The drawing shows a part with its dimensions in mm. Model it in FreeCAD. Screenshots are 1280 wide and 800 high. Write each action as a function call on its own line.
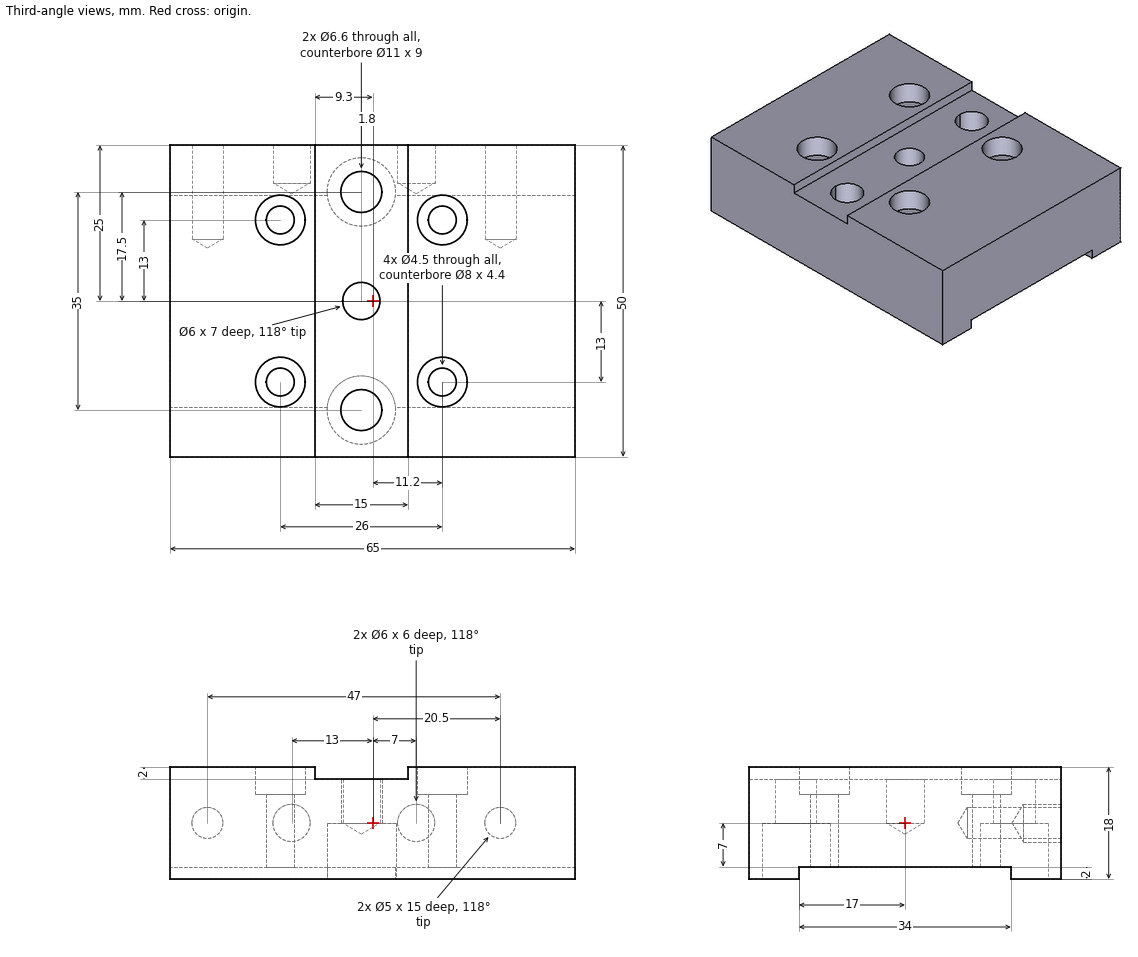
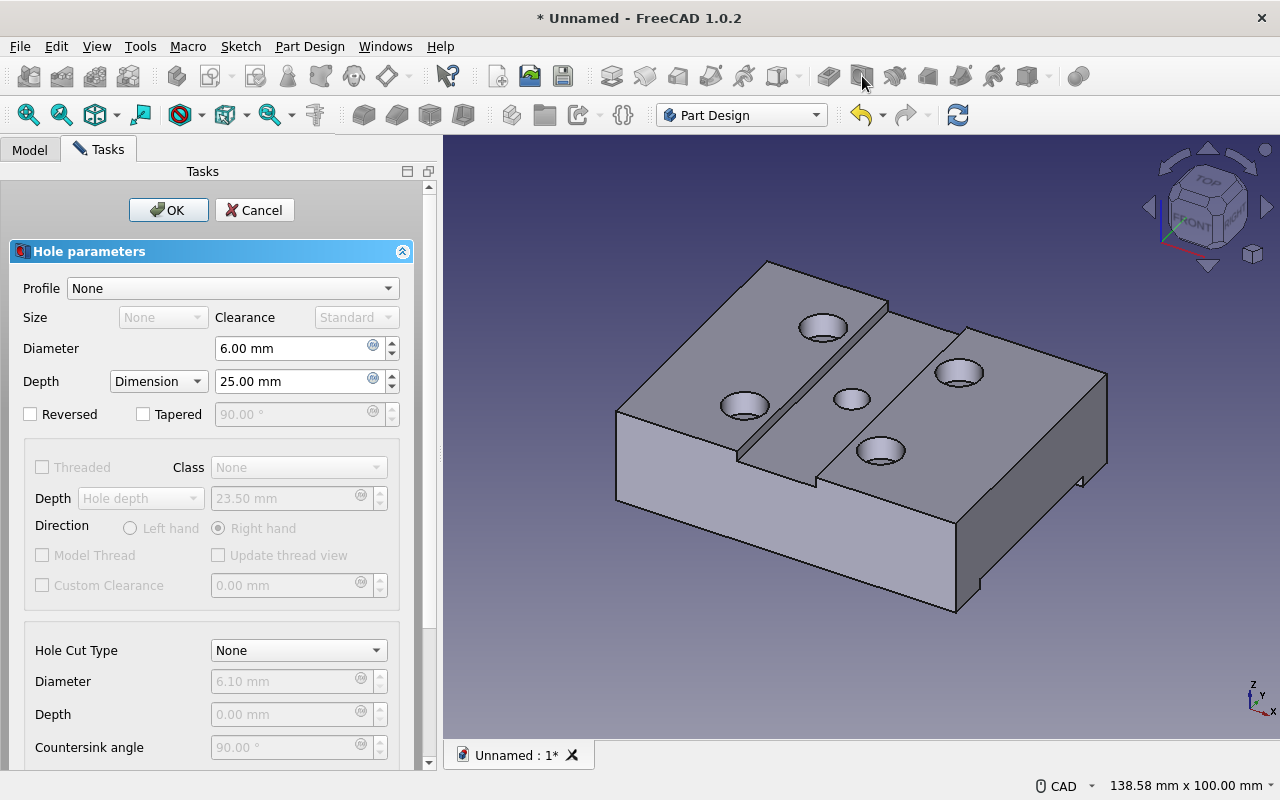
triple_click(300, 348)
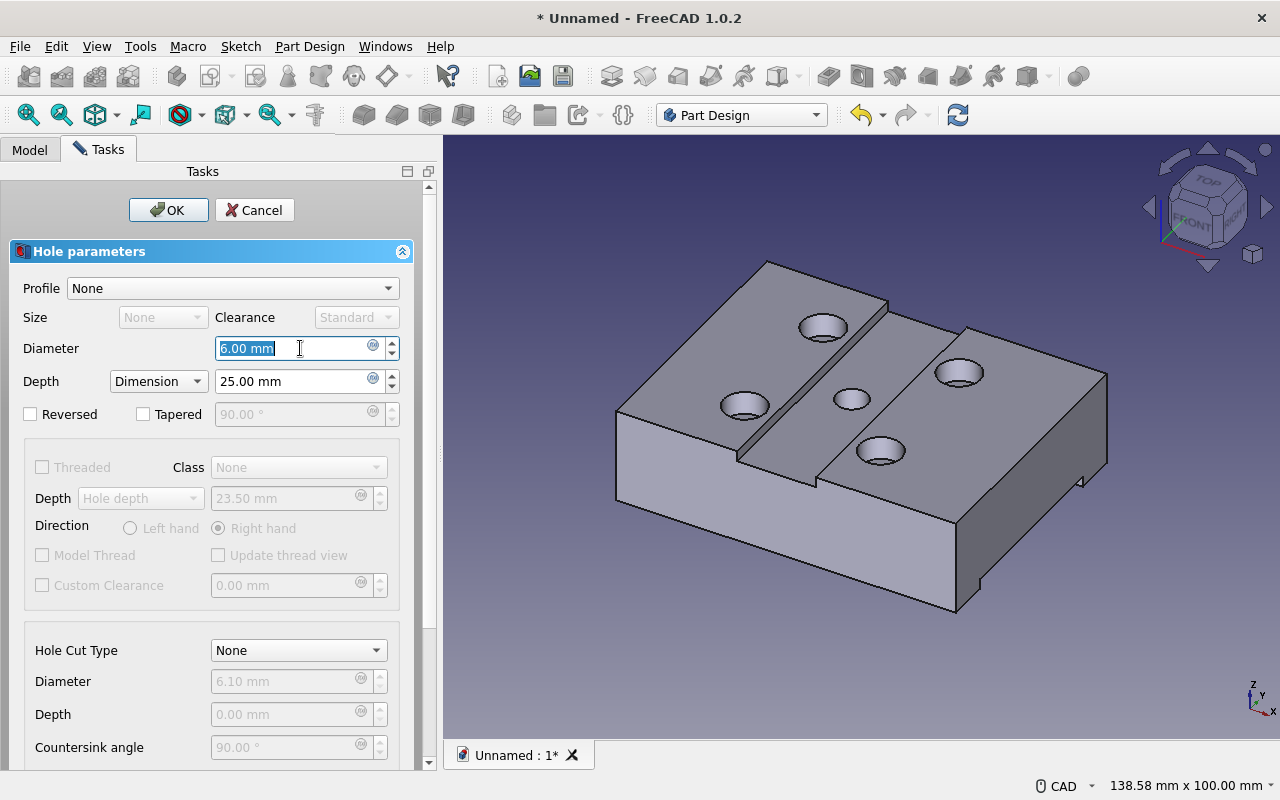
text(6)
key(Tab)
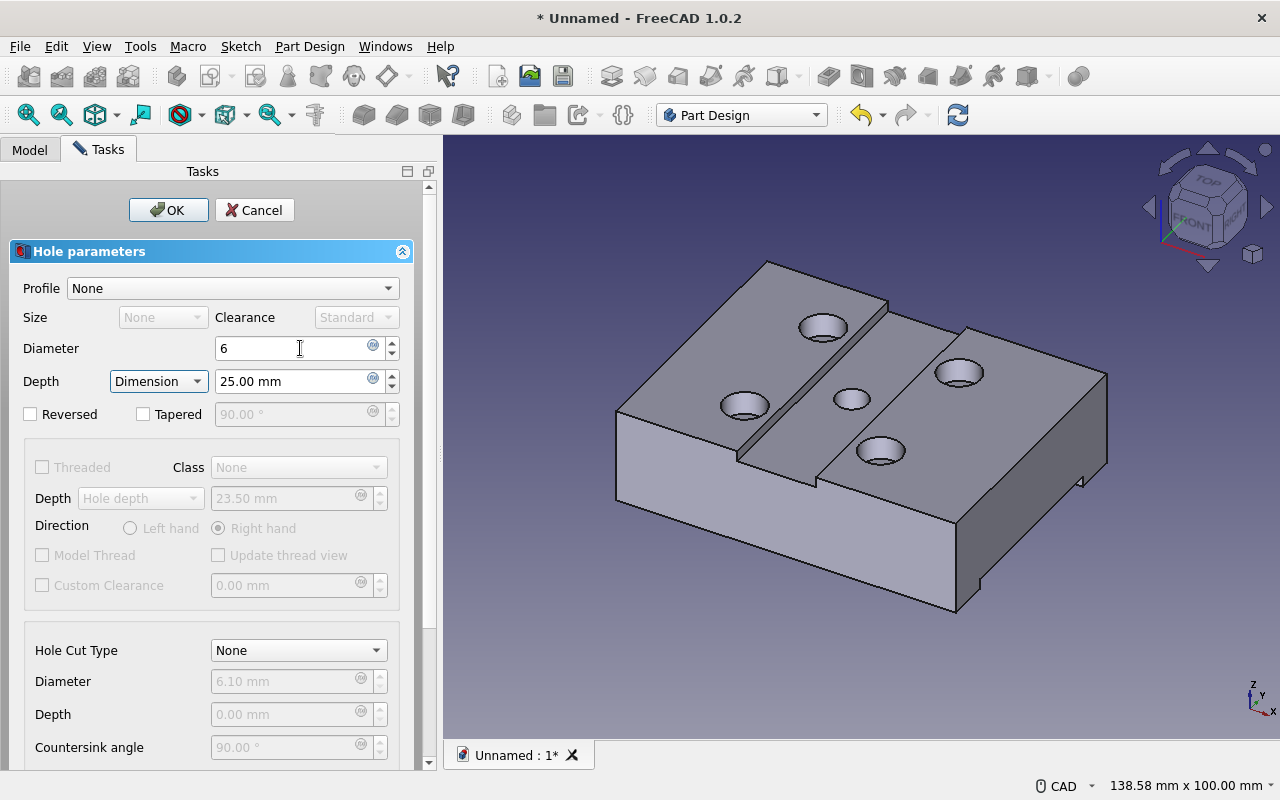
triple_click(300, 382)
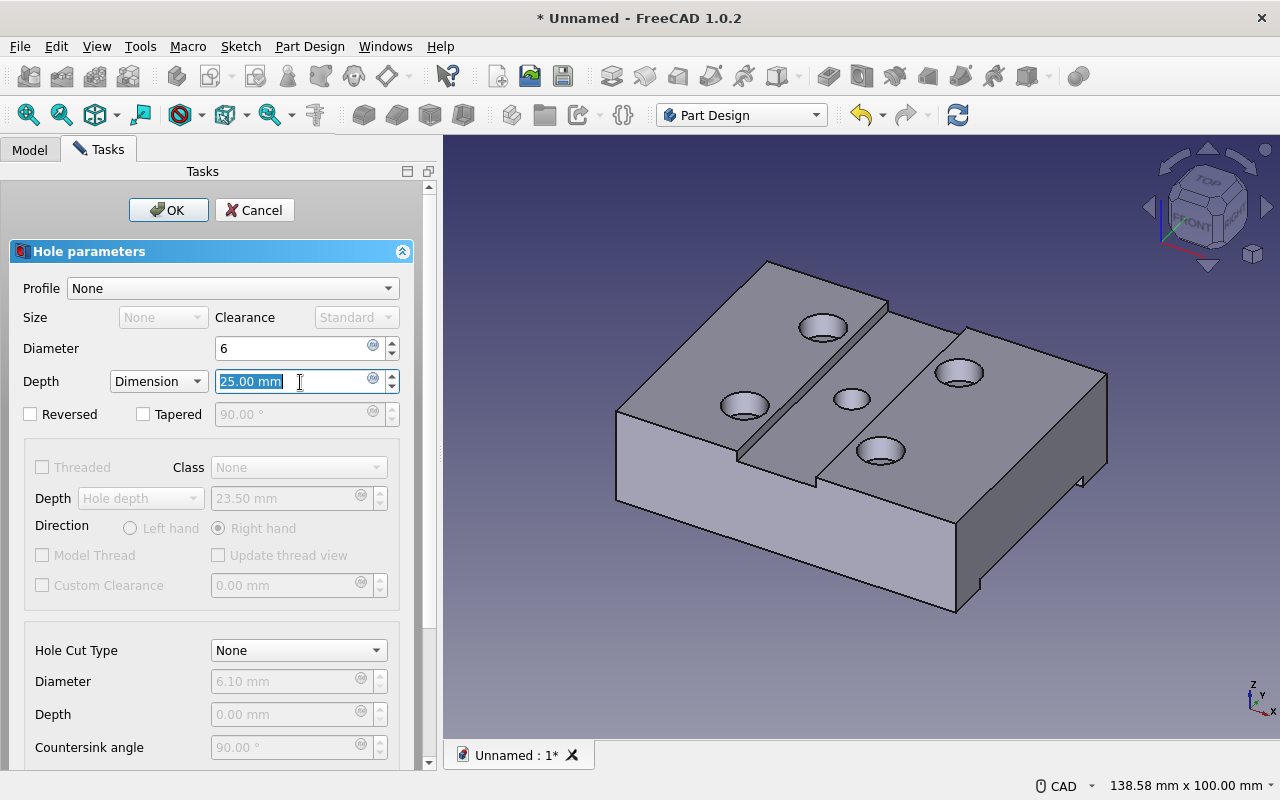
text(7)
key(Tab)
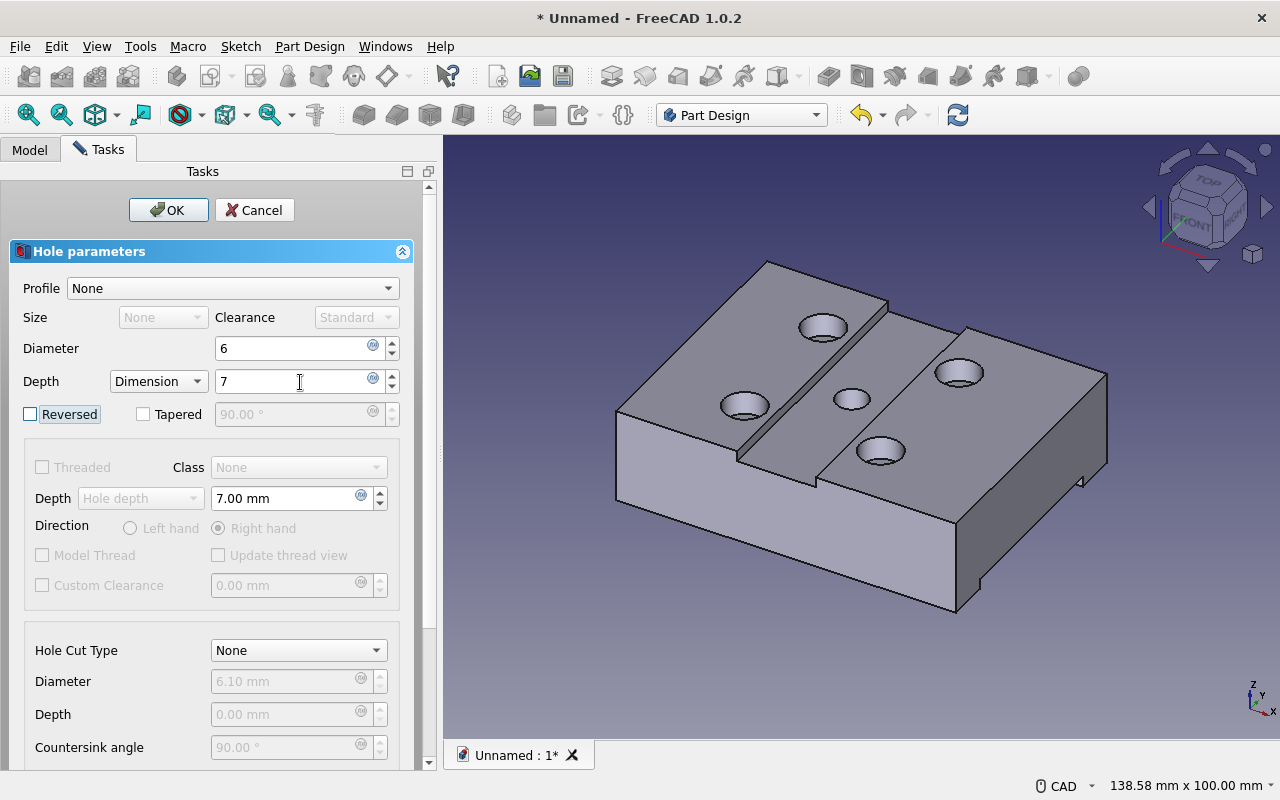
click(169, 210)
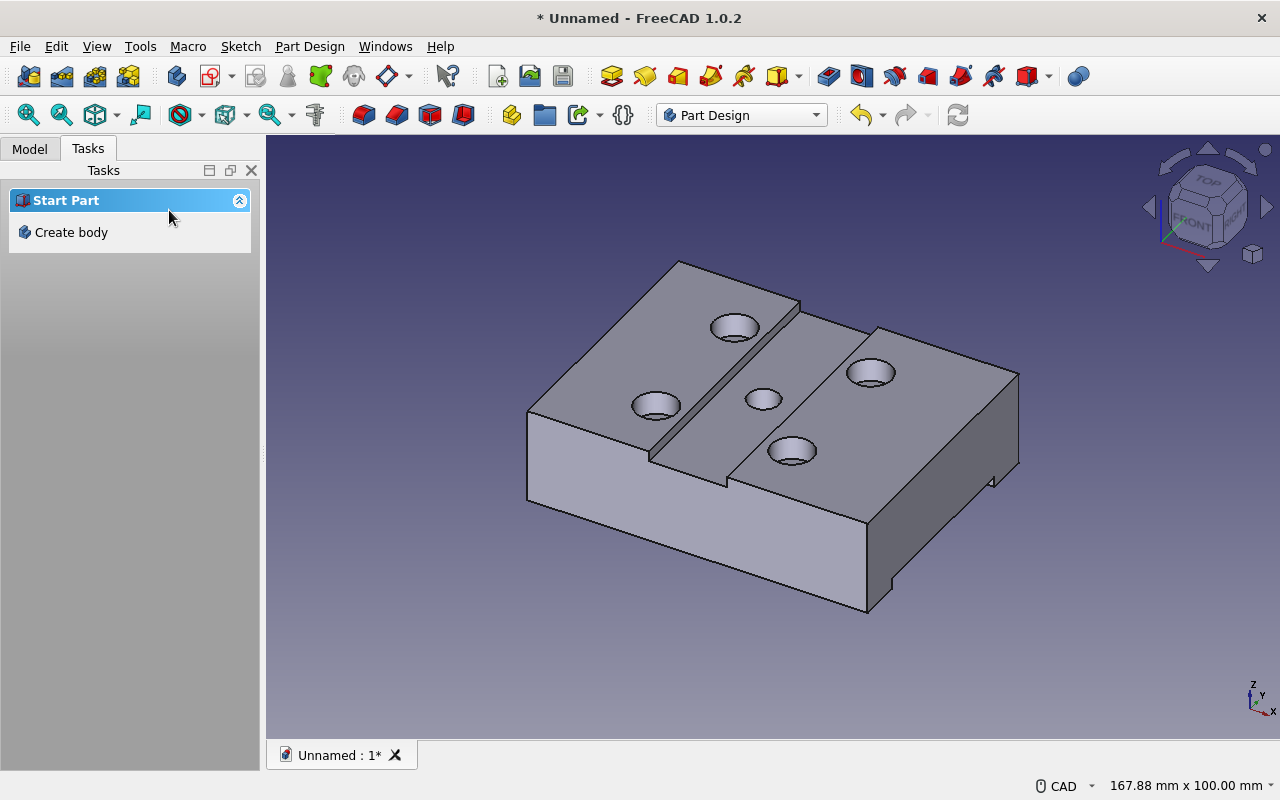
key(5)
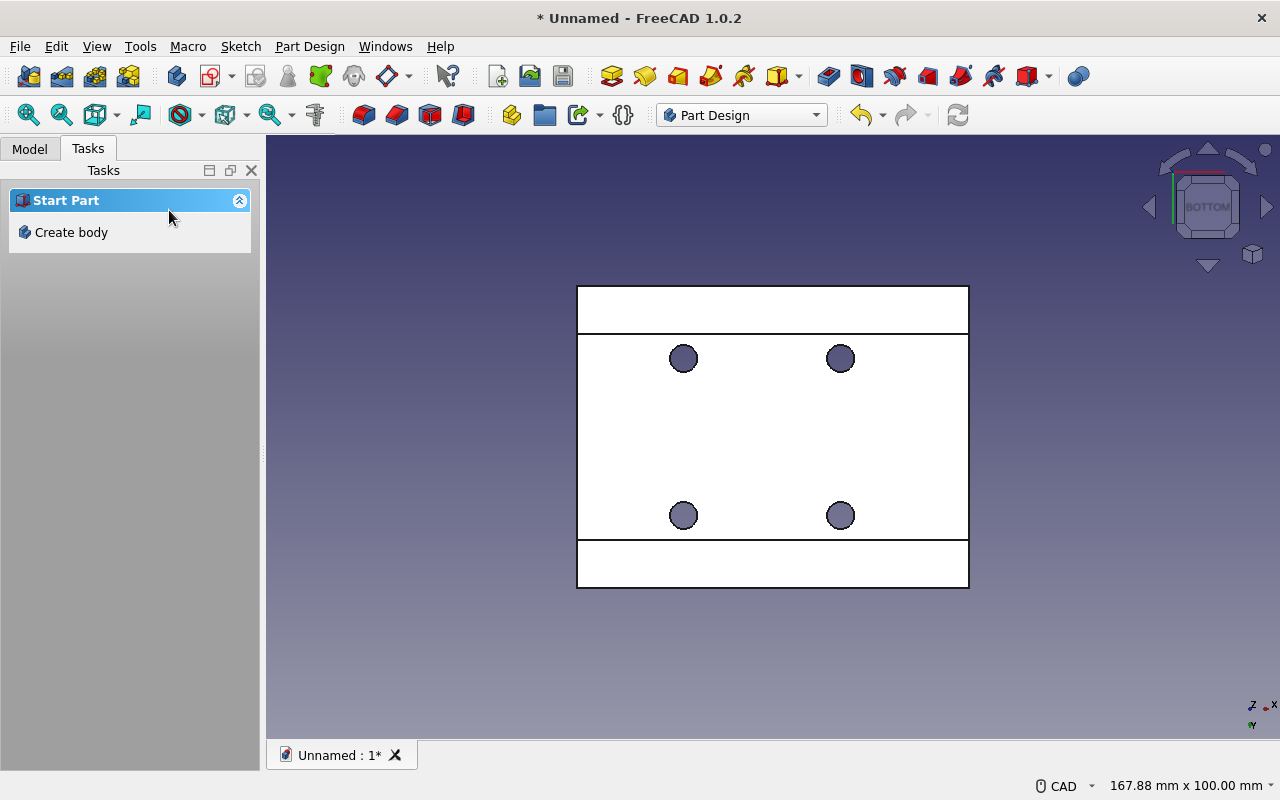
click(941, 309)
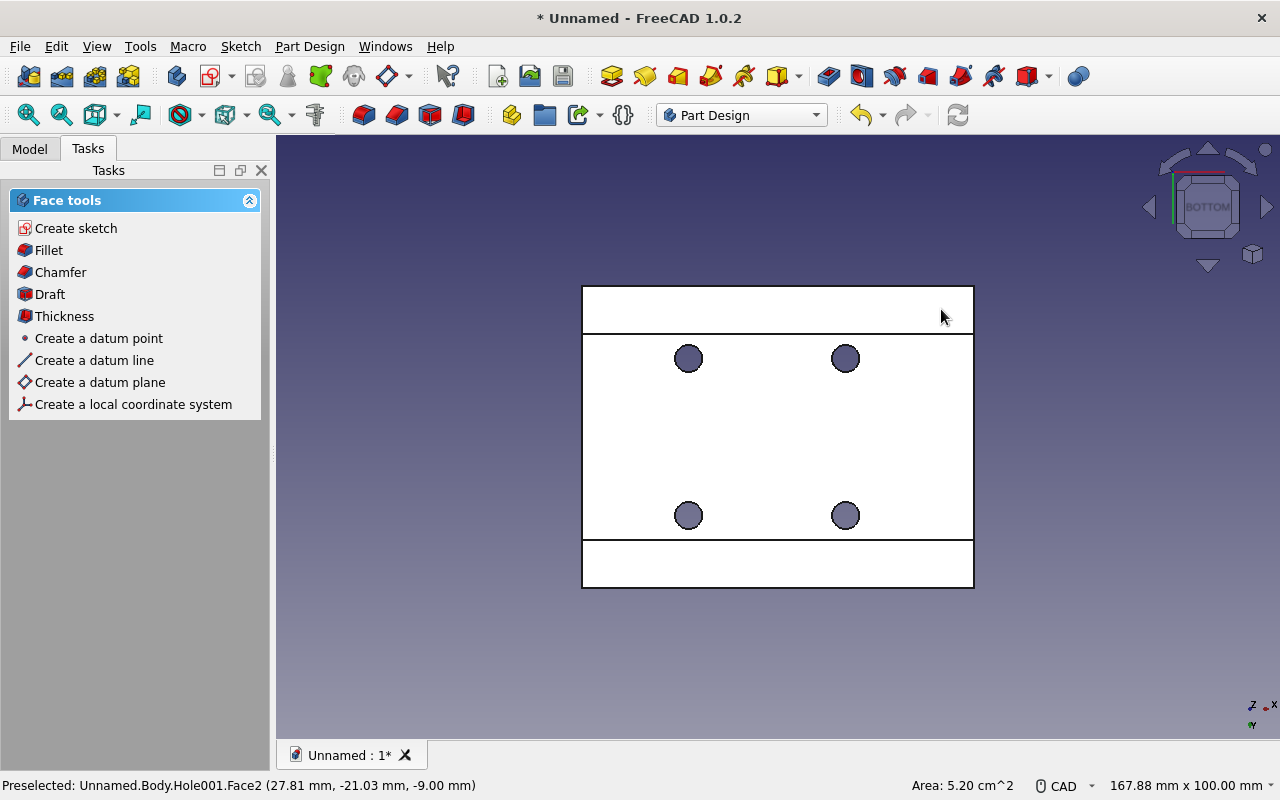
click(210, 76)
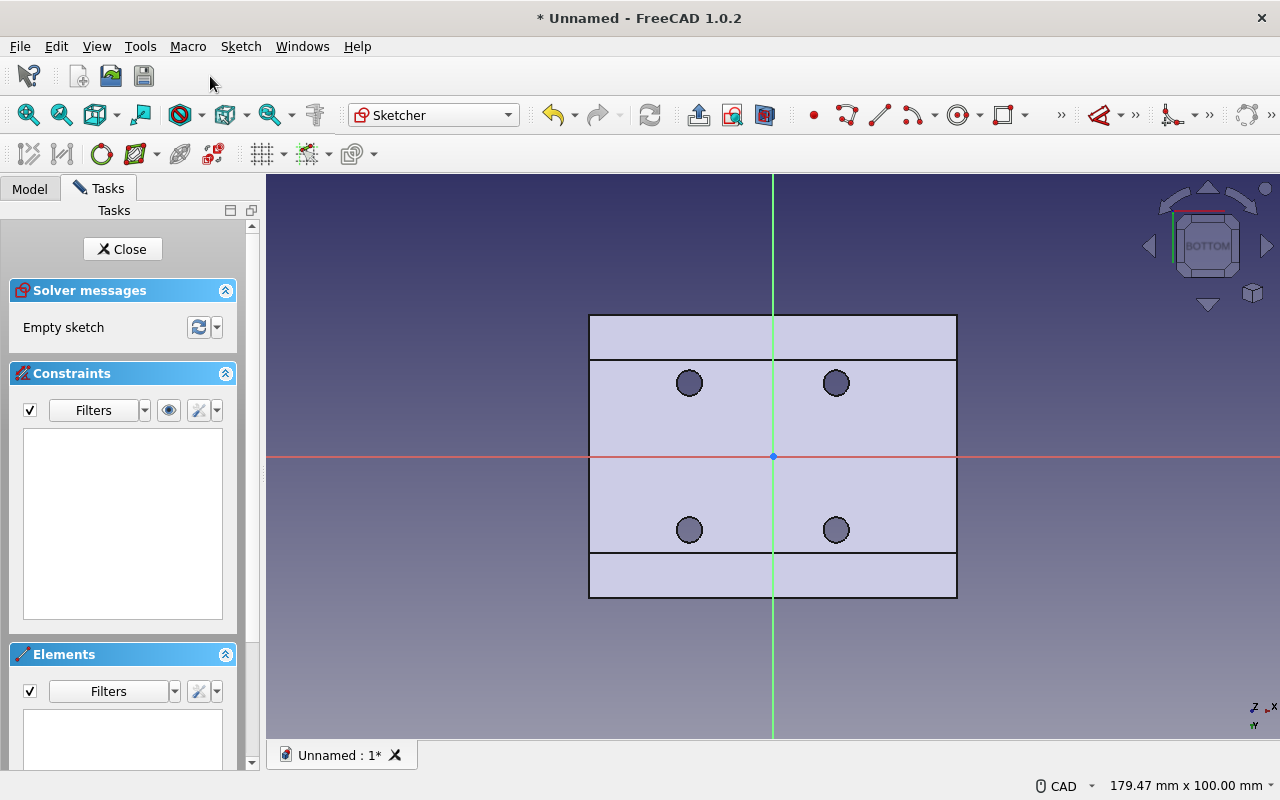
scroll(881, 456, up, 2)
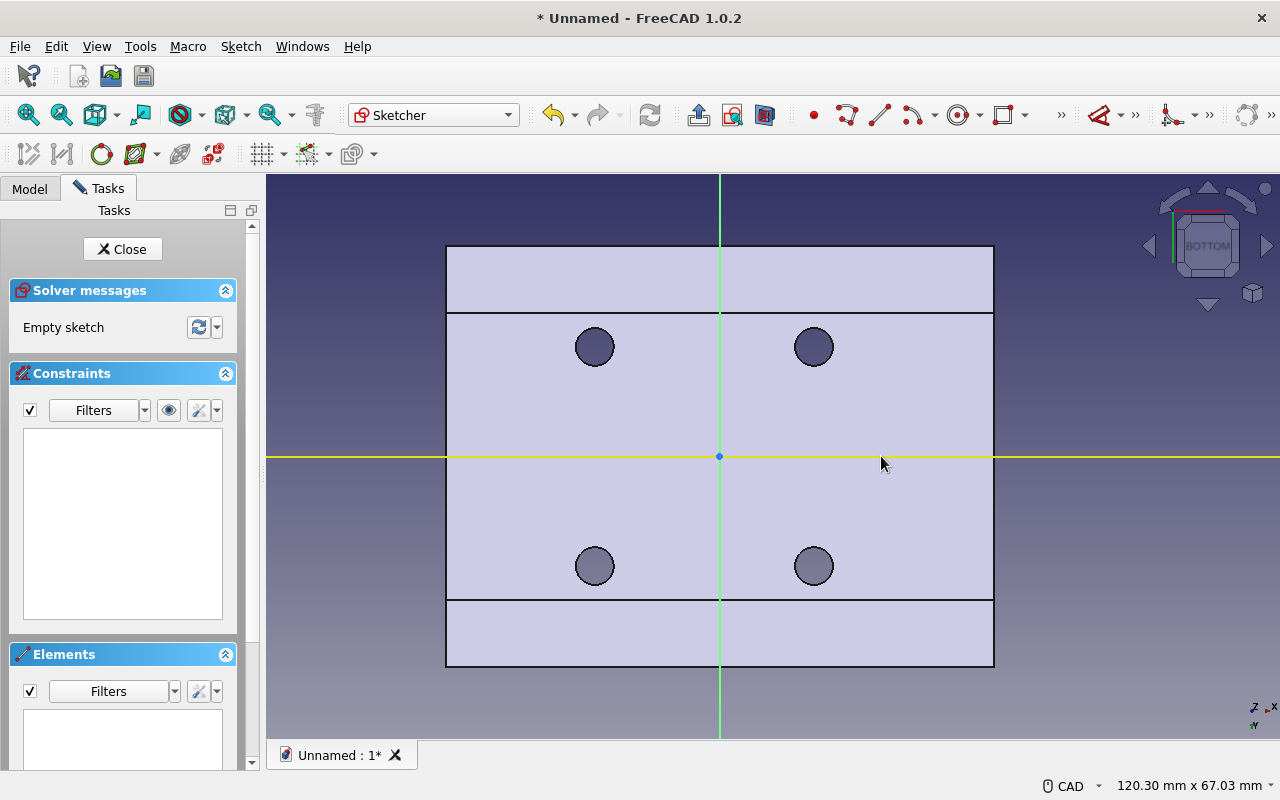
click(958, 116)